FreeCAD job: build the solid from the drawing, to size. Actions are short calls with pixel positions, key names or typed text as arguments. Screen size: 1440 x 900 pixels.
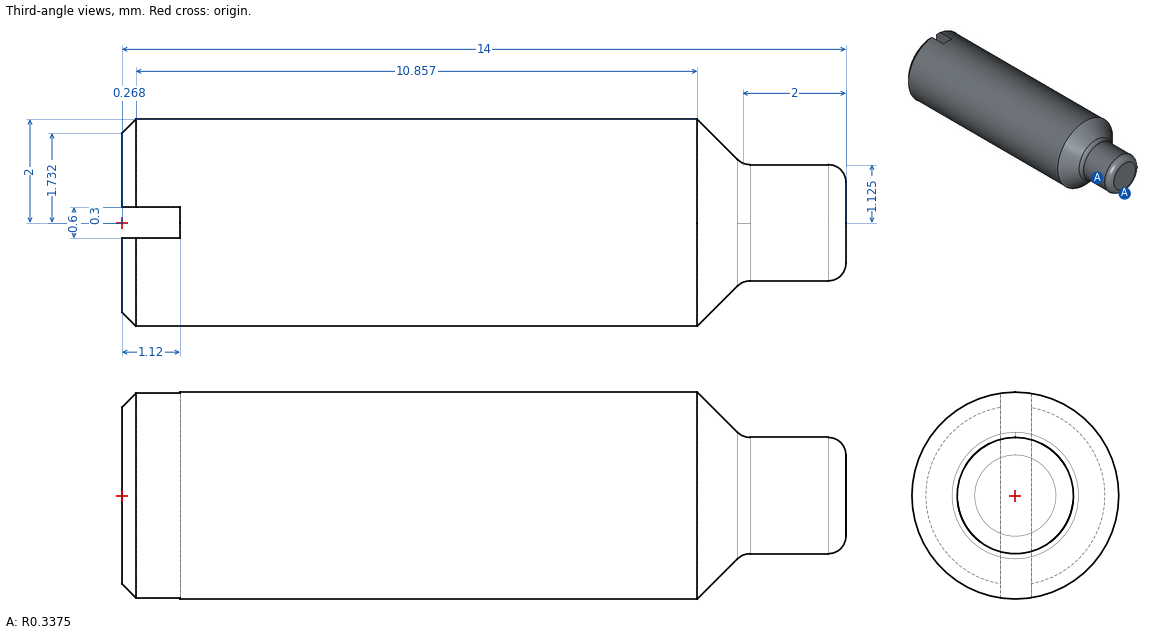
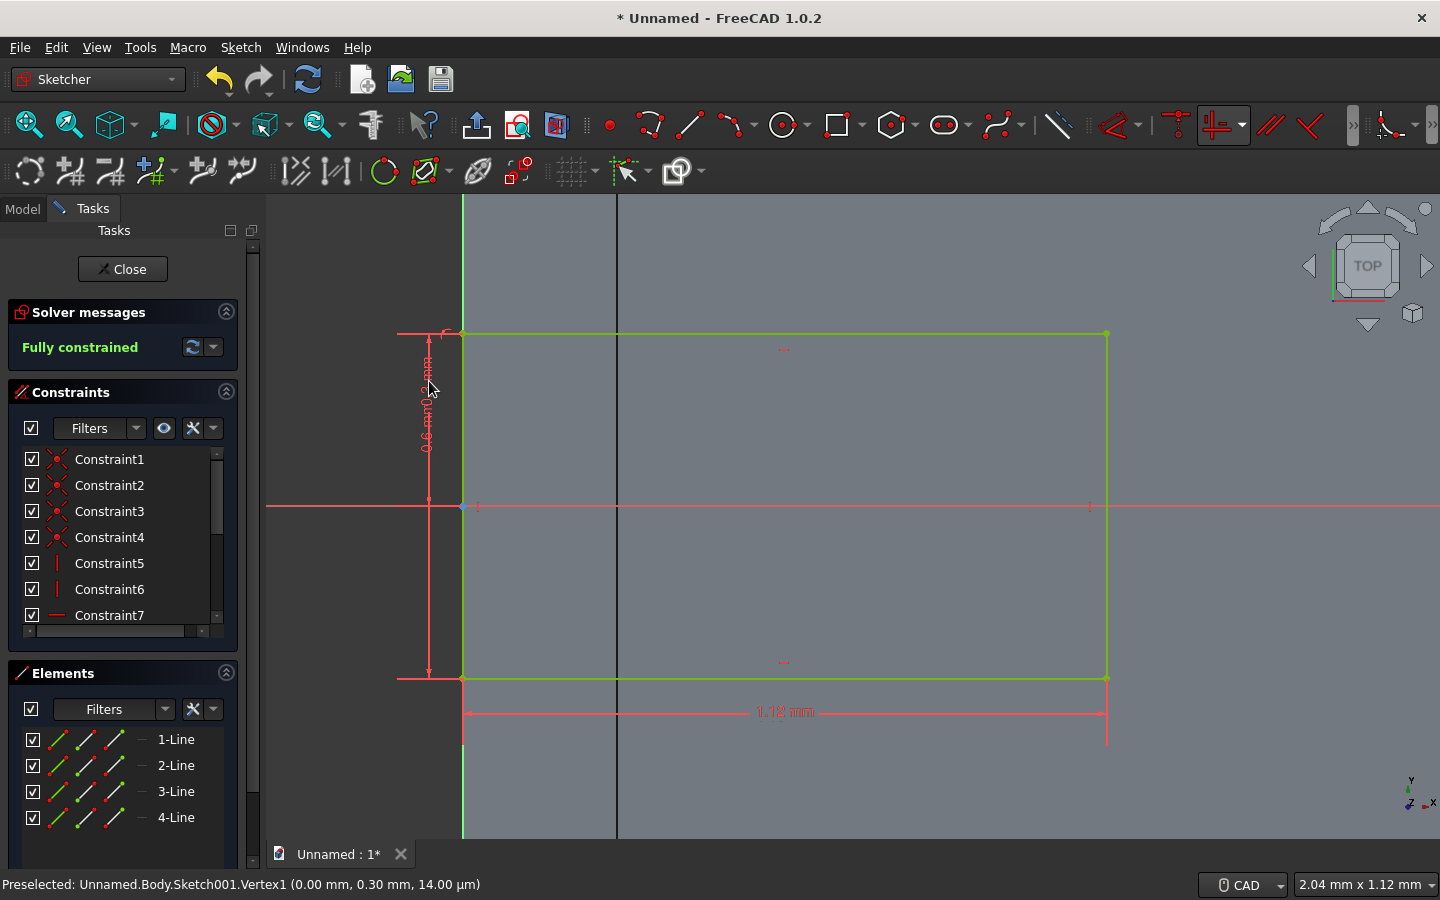
click(123, 269)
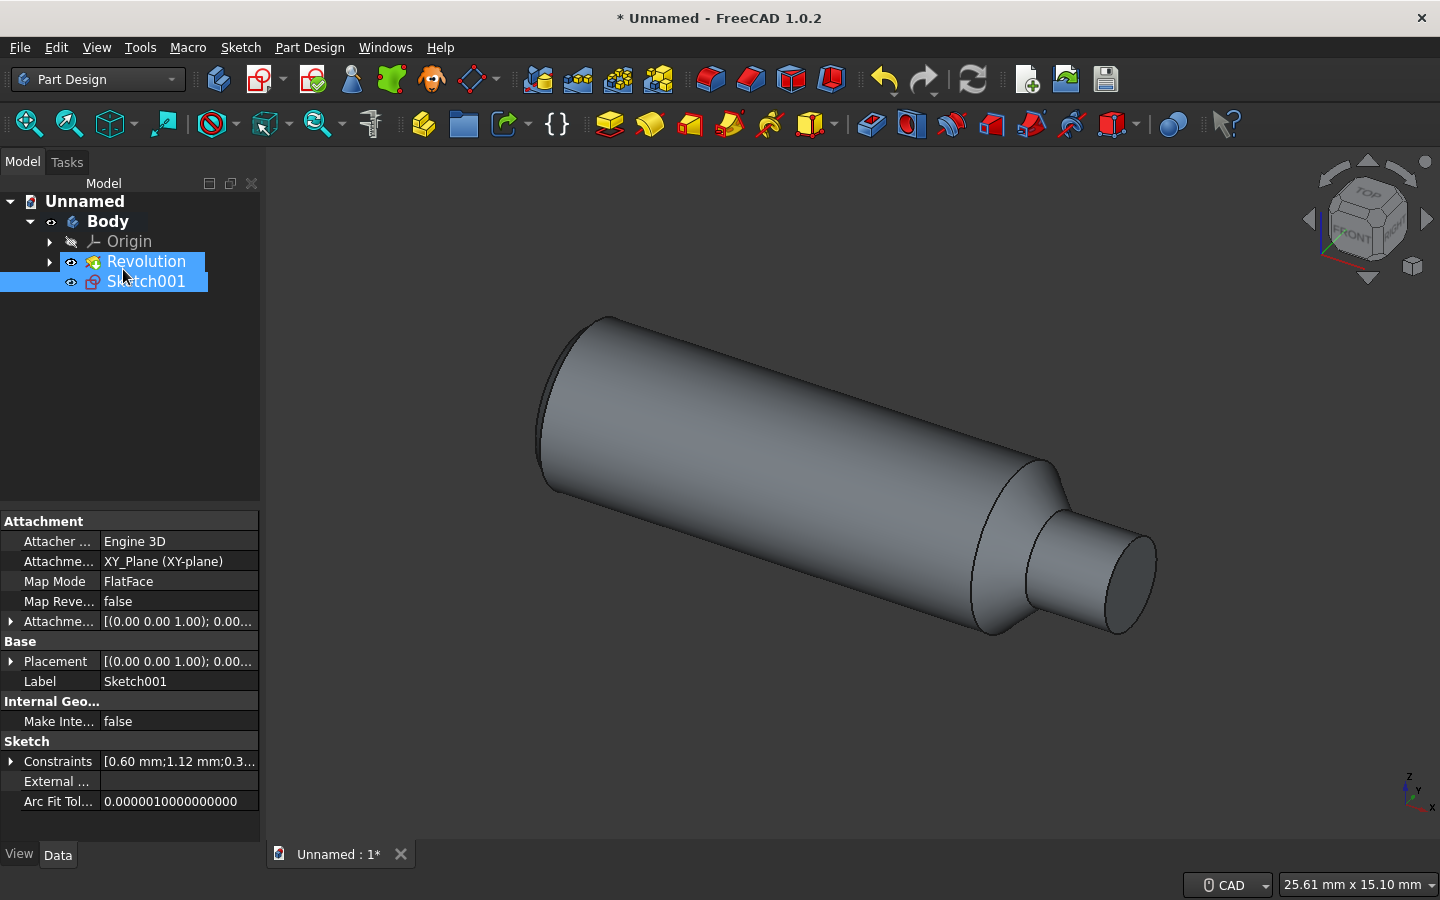
click(872, 124)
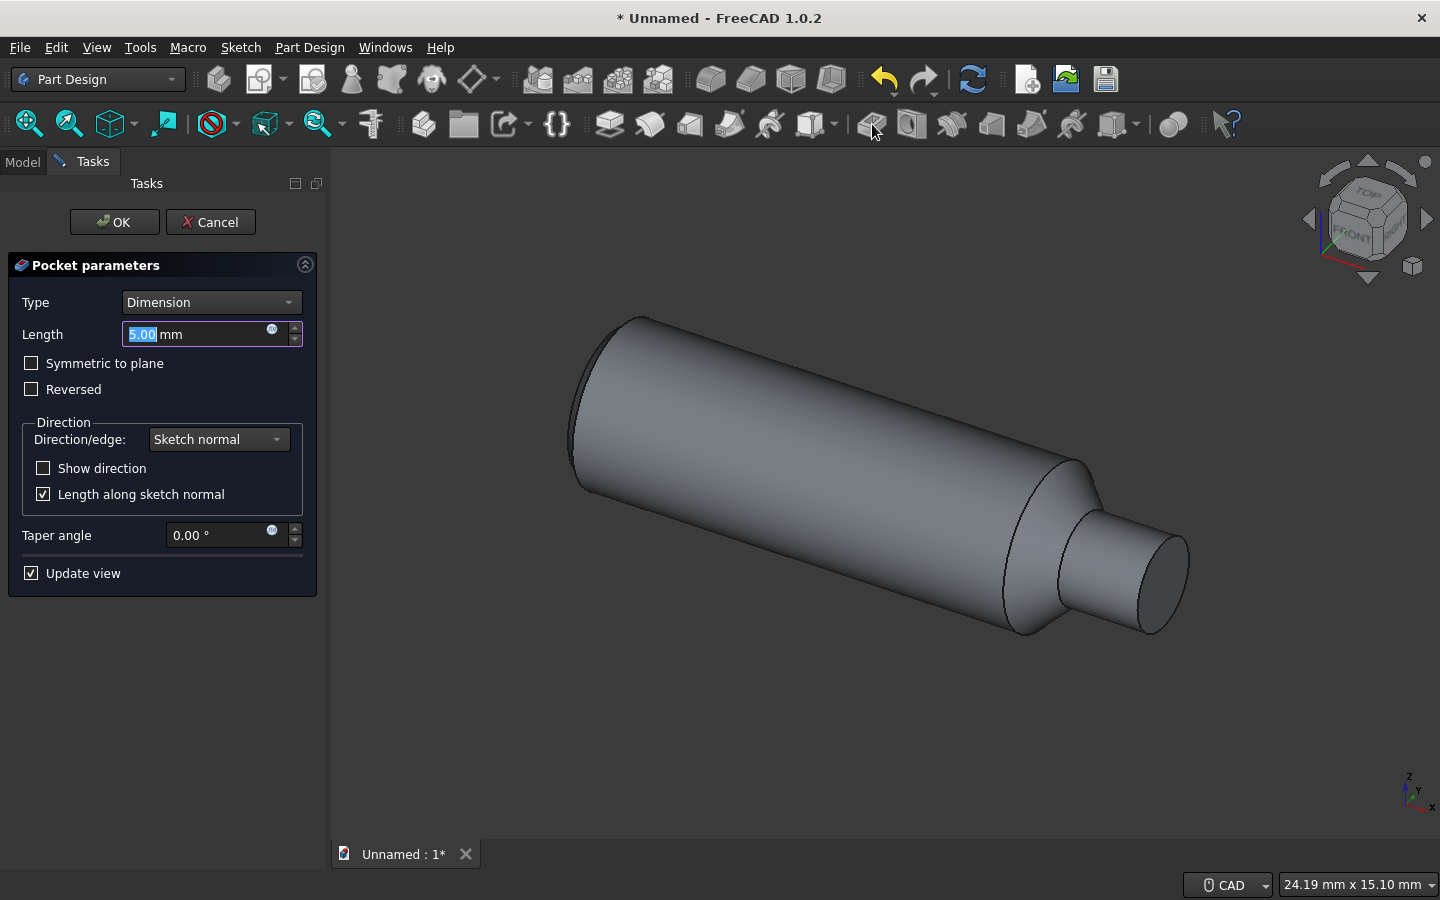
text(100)
key(Tab)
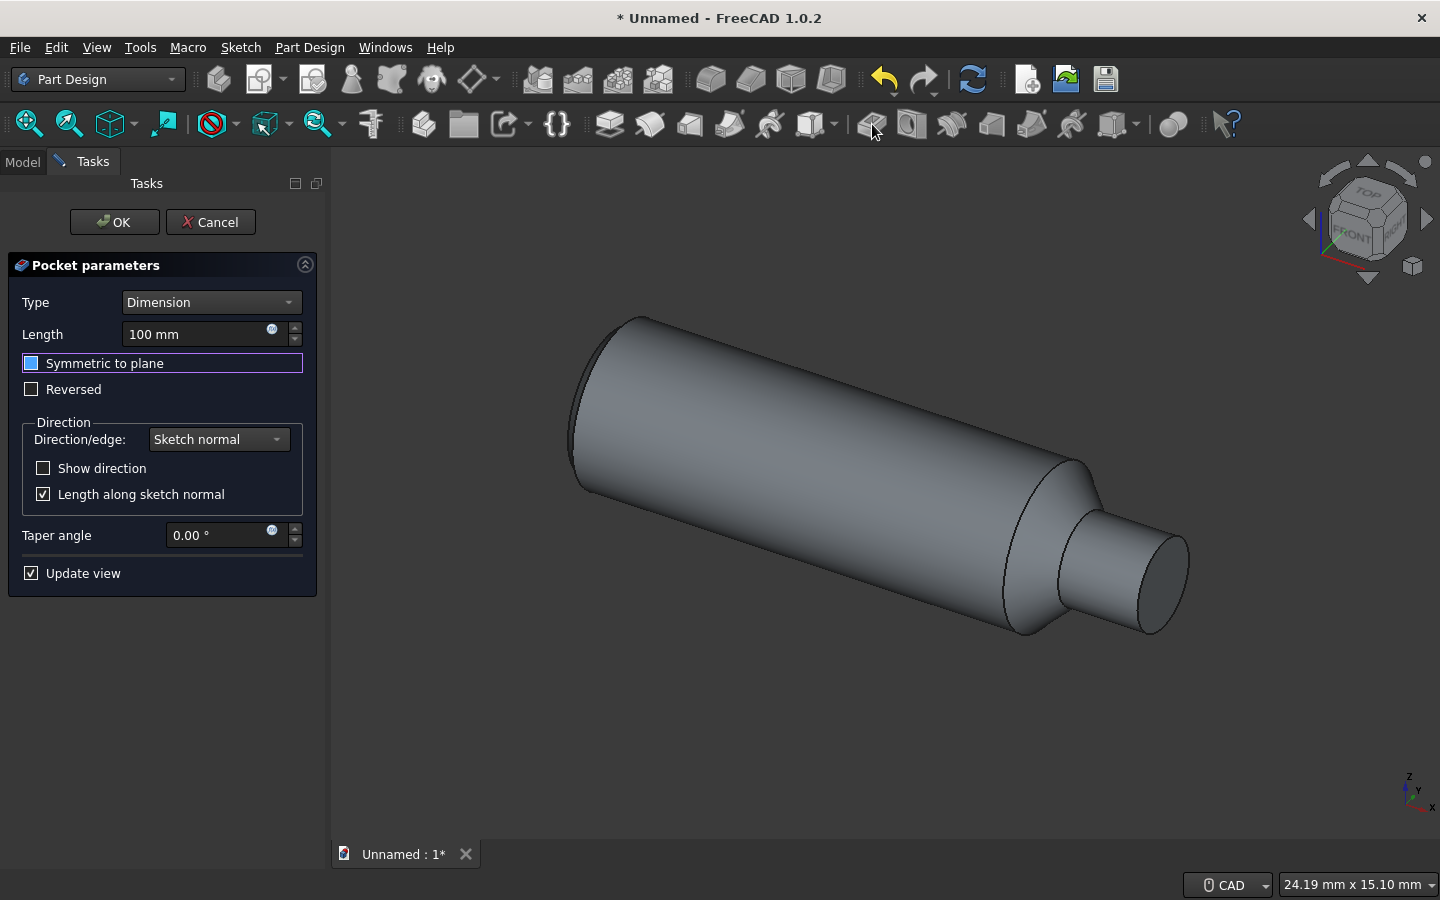
click(30, 363)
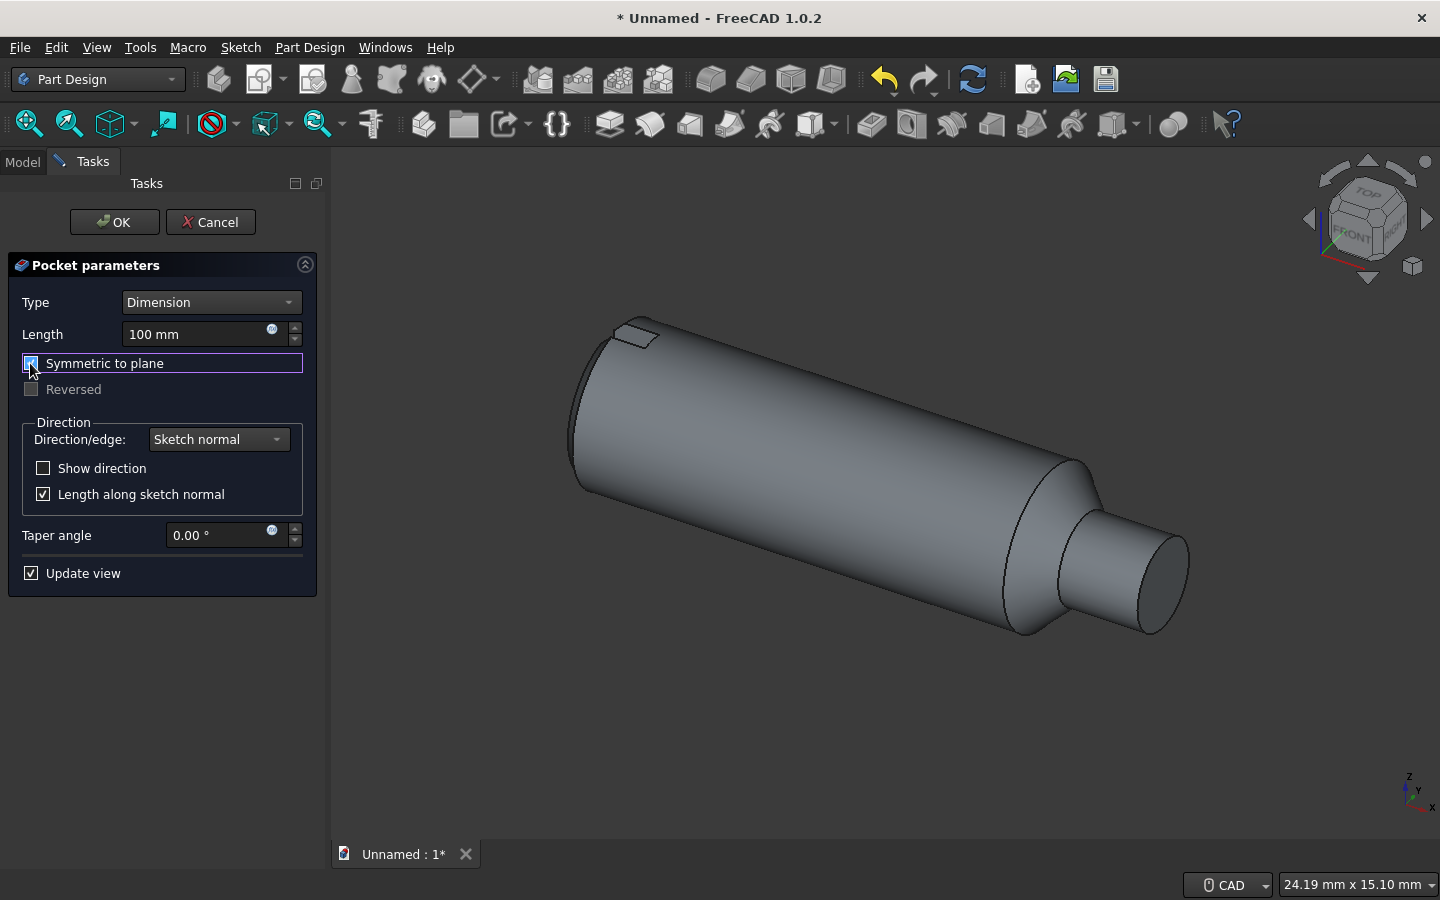
click(115, 222)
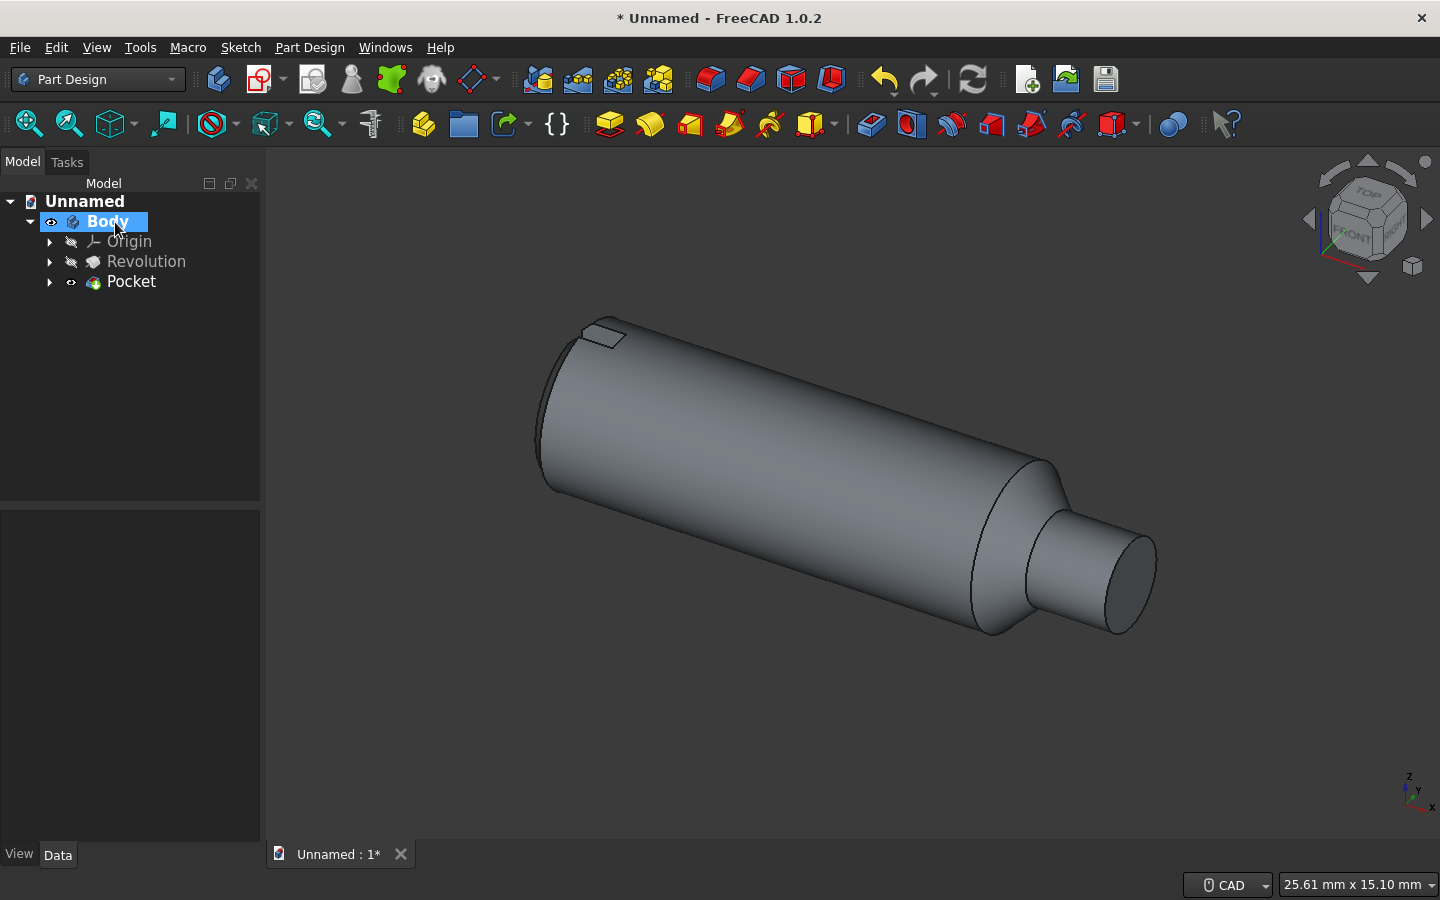
click(1105, 610)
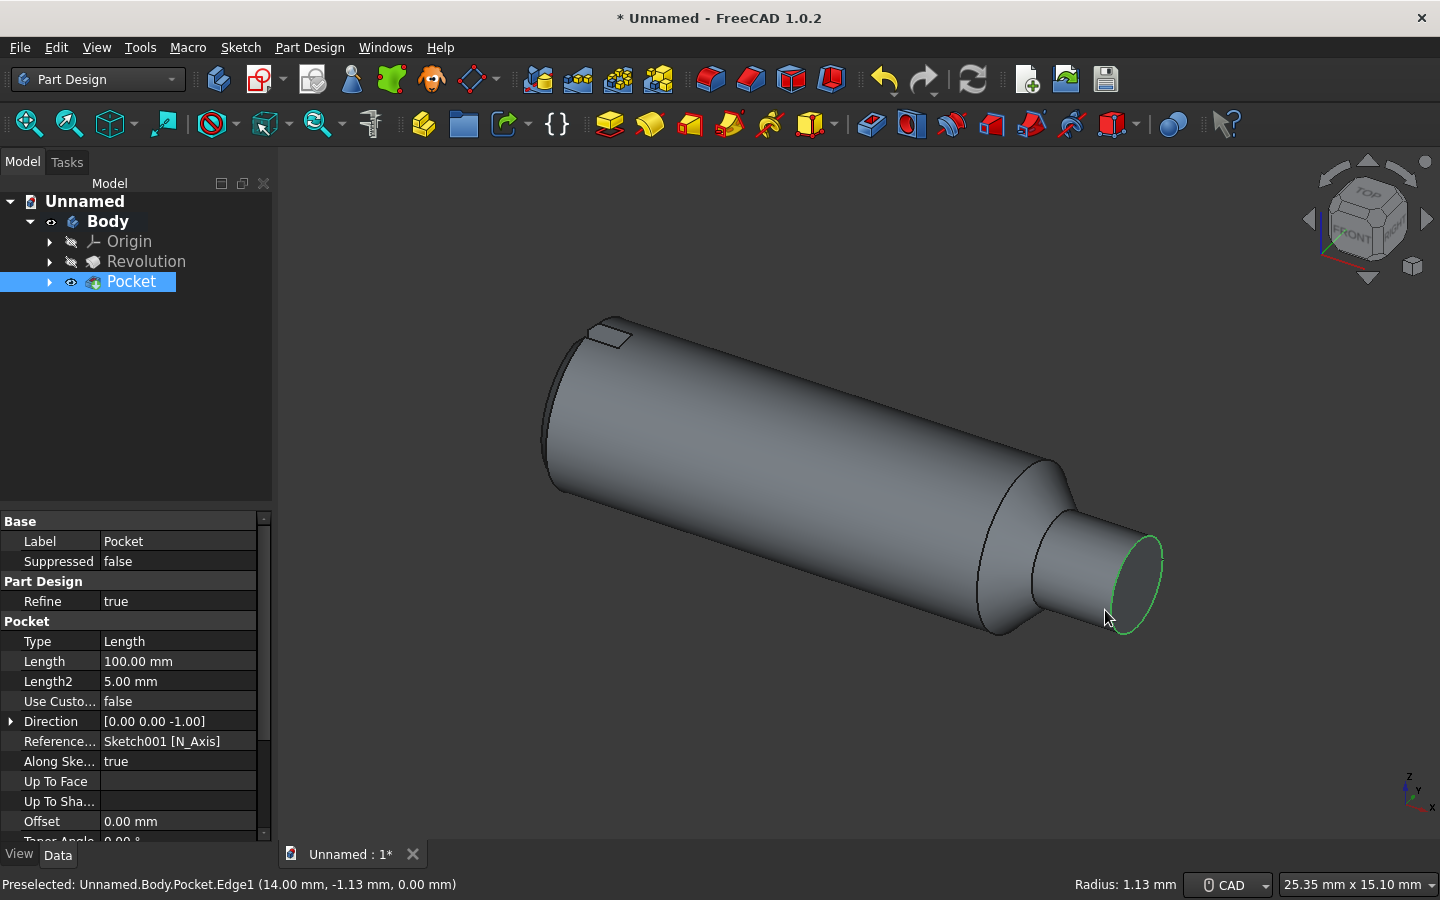
click(1065, 510, ctrl)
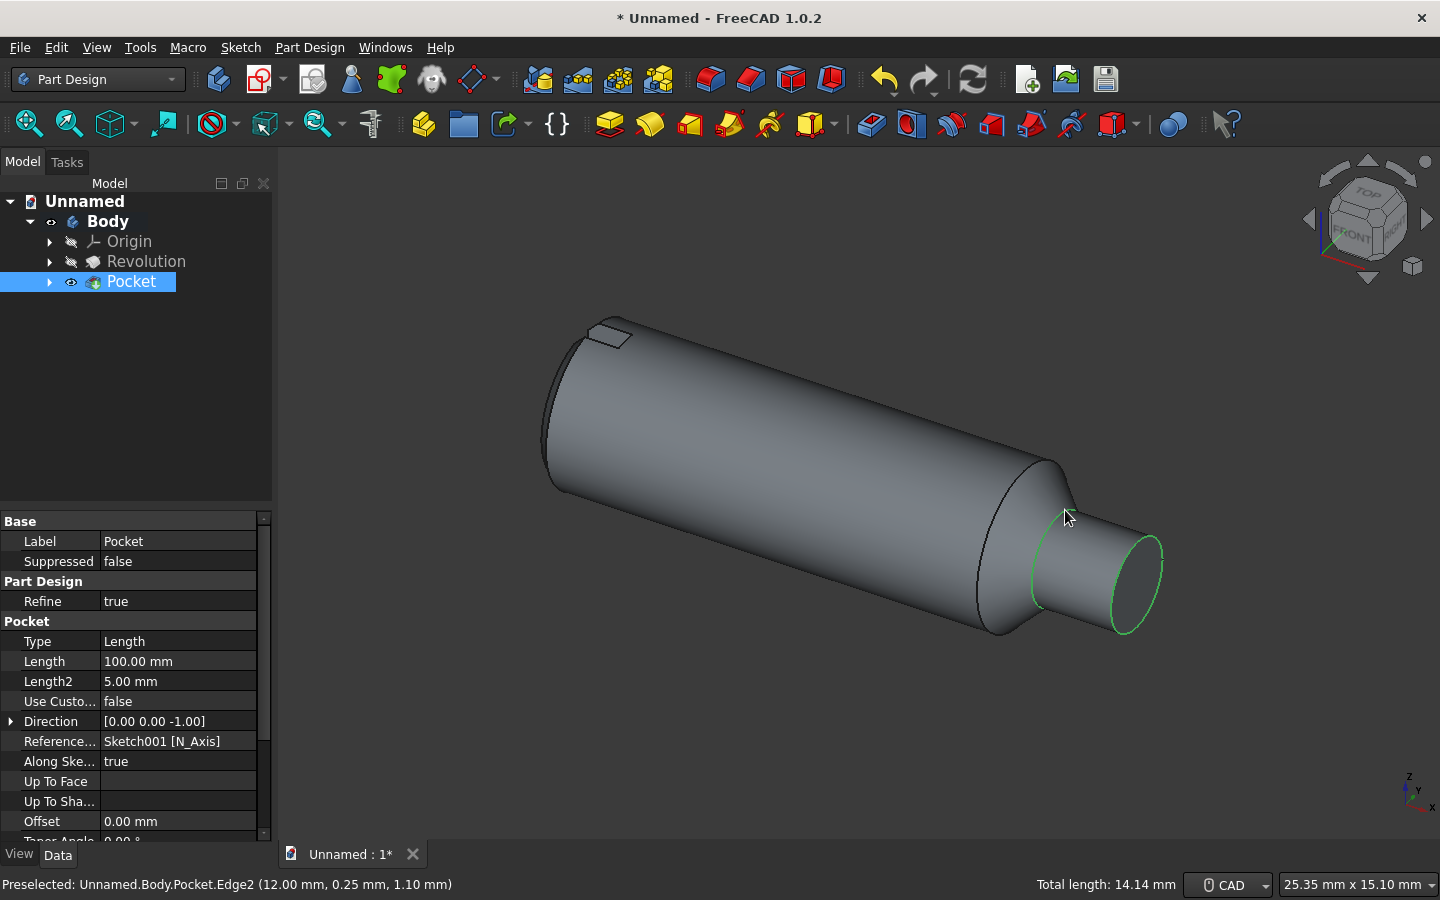
click(712, 80)